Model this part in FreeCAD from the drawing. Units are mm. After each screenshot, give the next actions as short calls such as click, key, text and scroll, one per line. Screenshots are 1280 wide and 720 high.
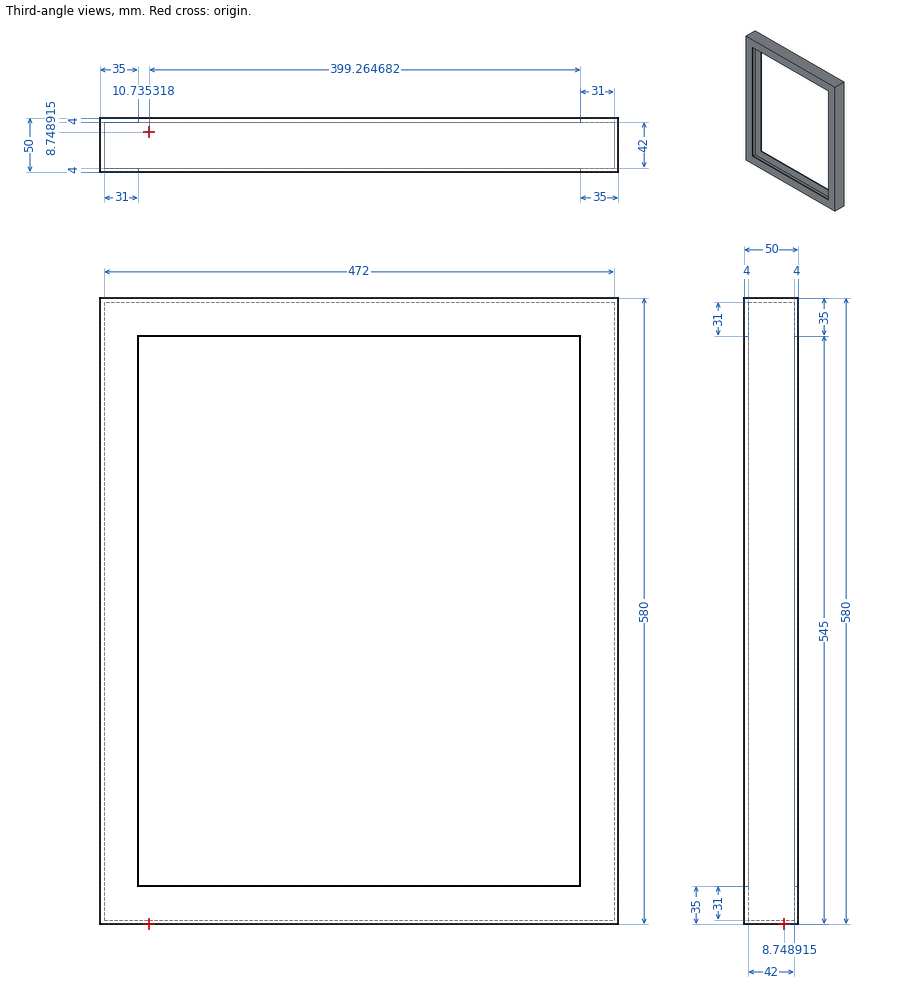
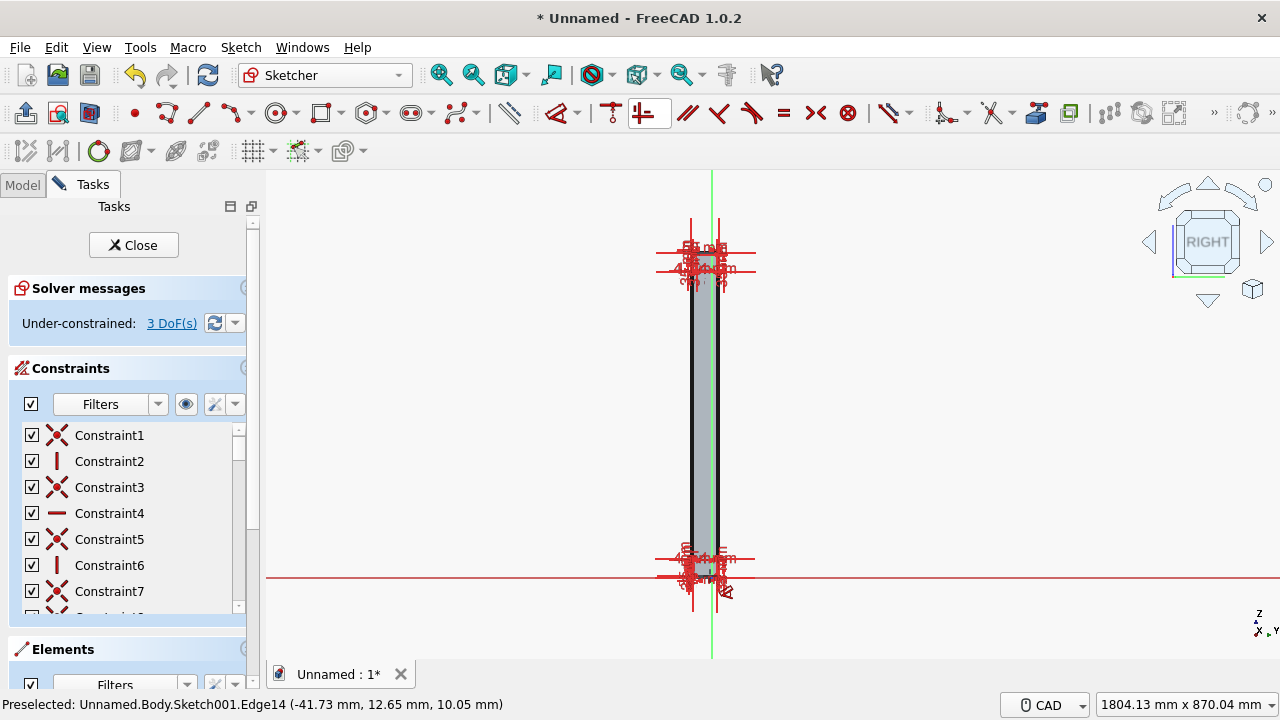
scroll(717, 272, up, 9)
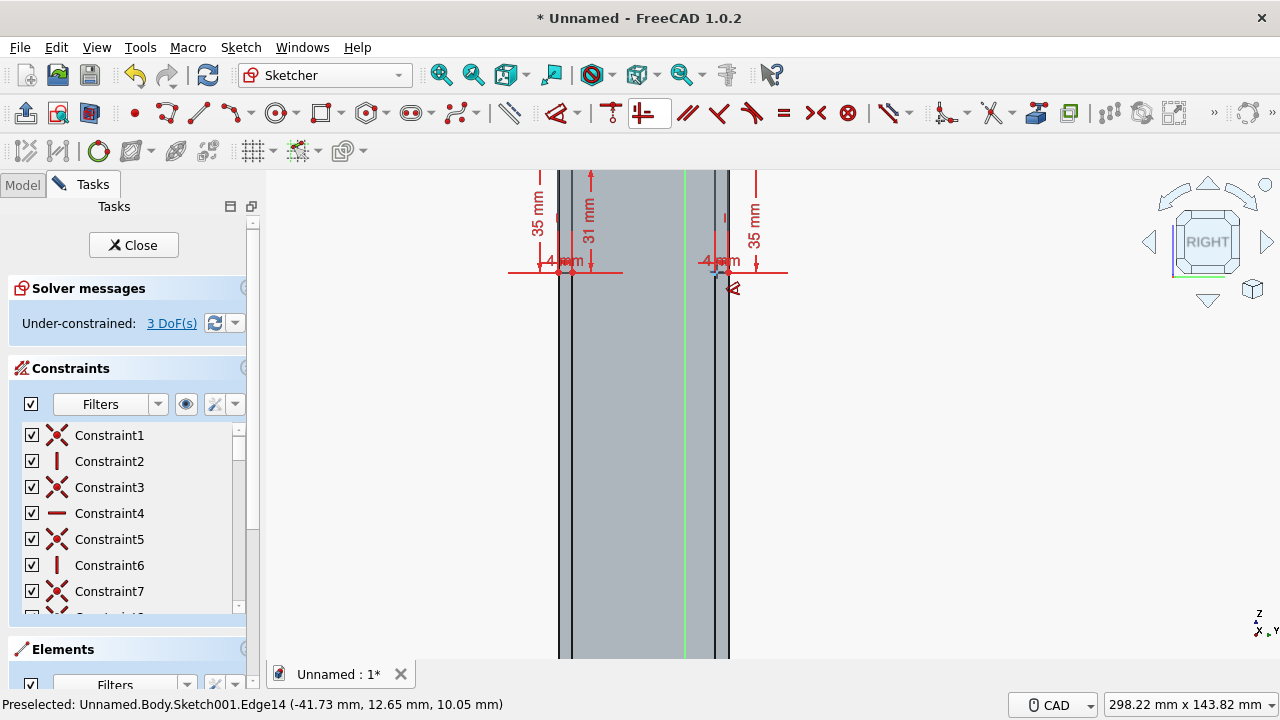
click(715, 273)
click(749, 452)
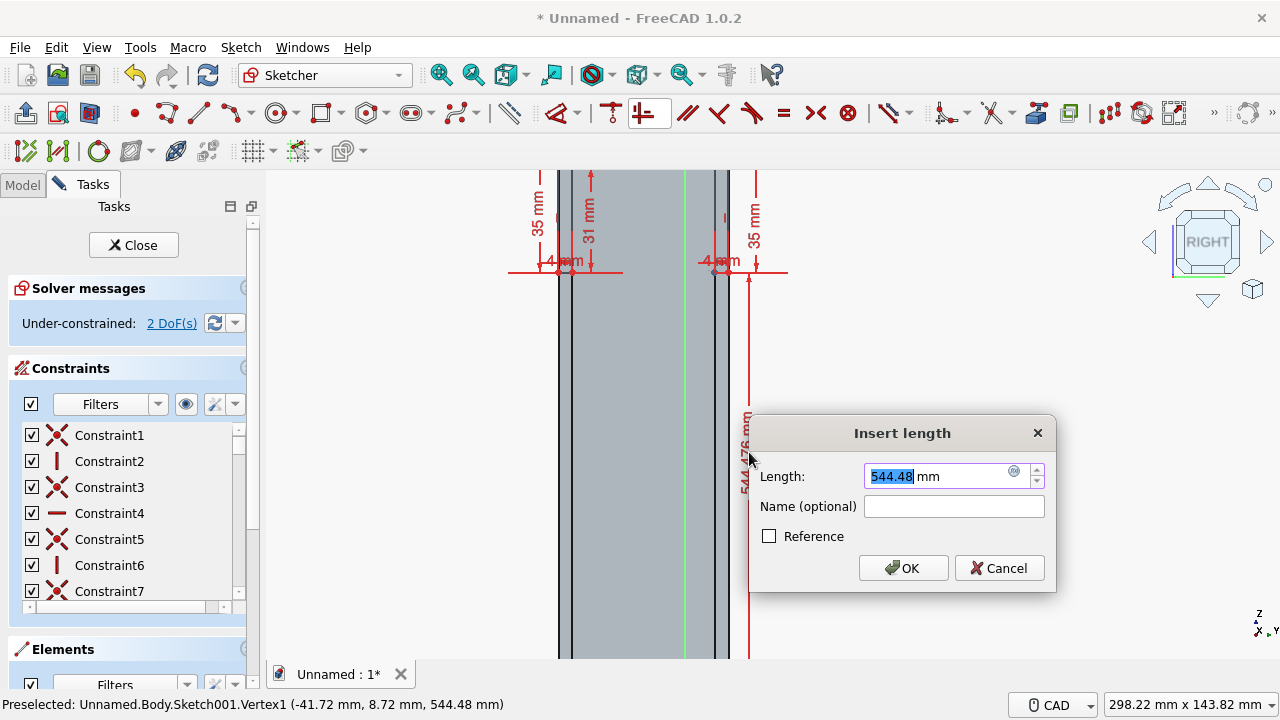
text(545)
key(Return)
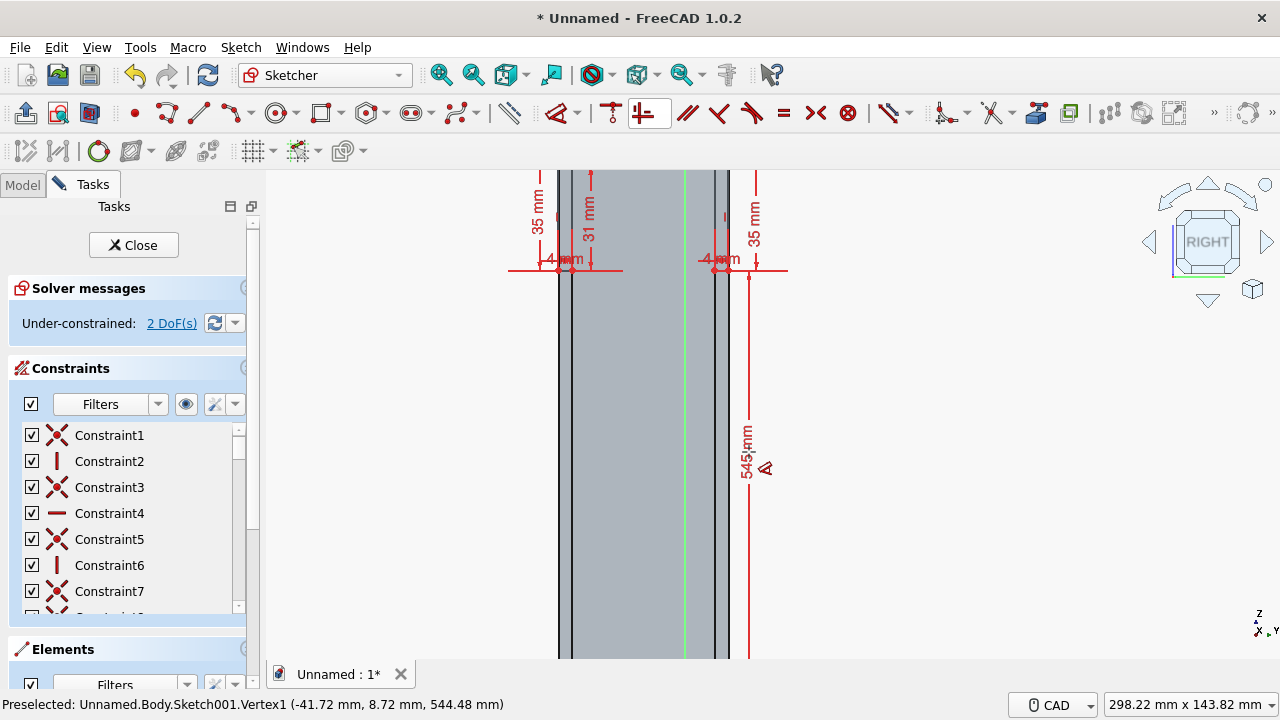
scroll(715, 271, up, 2)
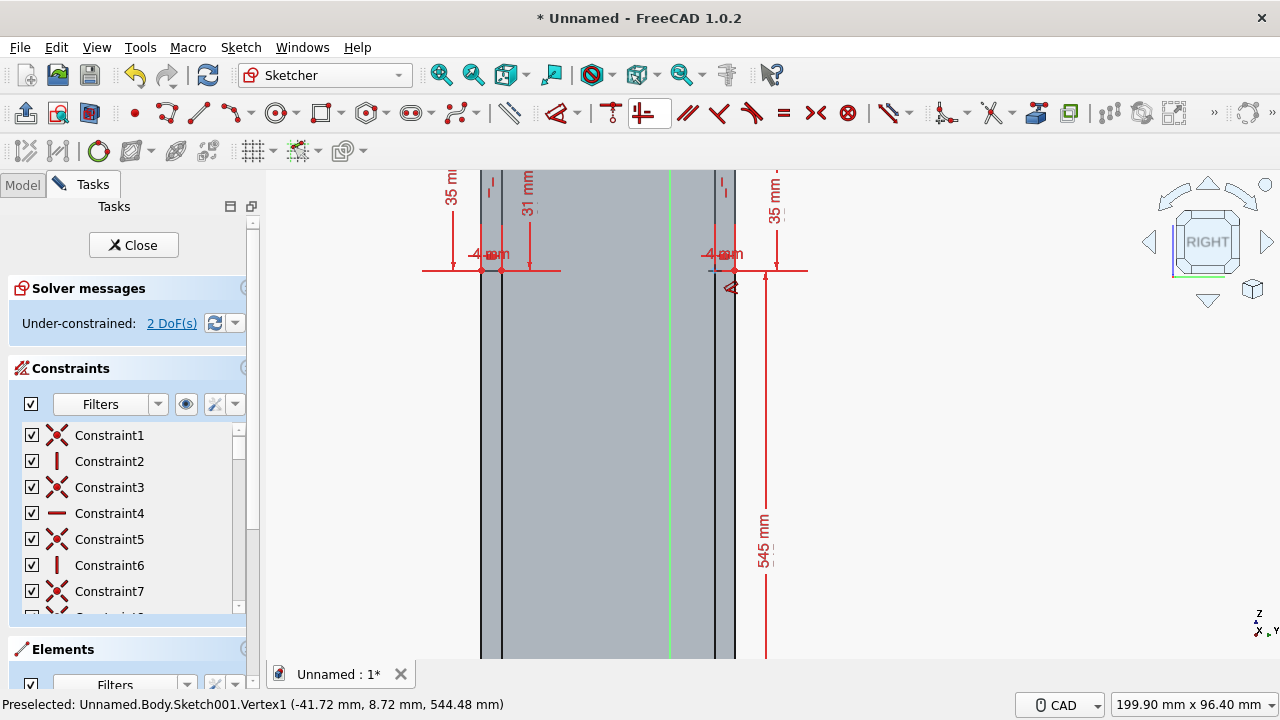
click(715, 271)
click(693, 237)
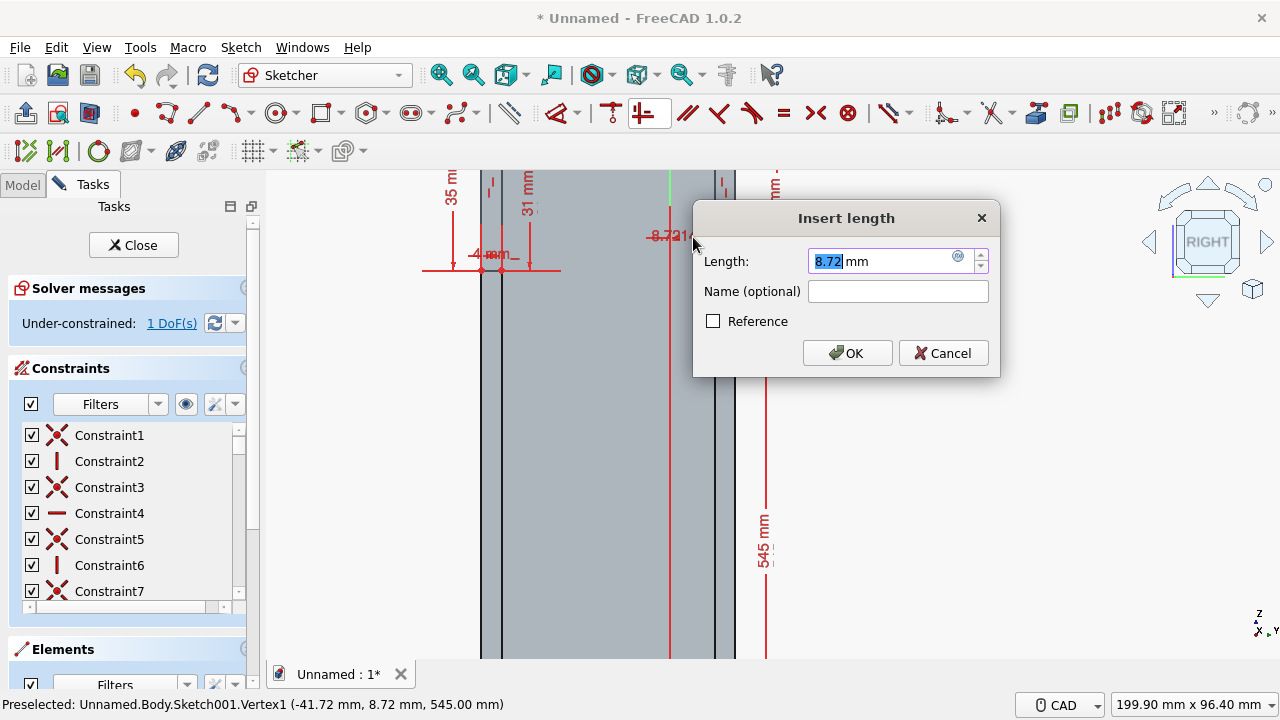
text(8.748915)
key(Return)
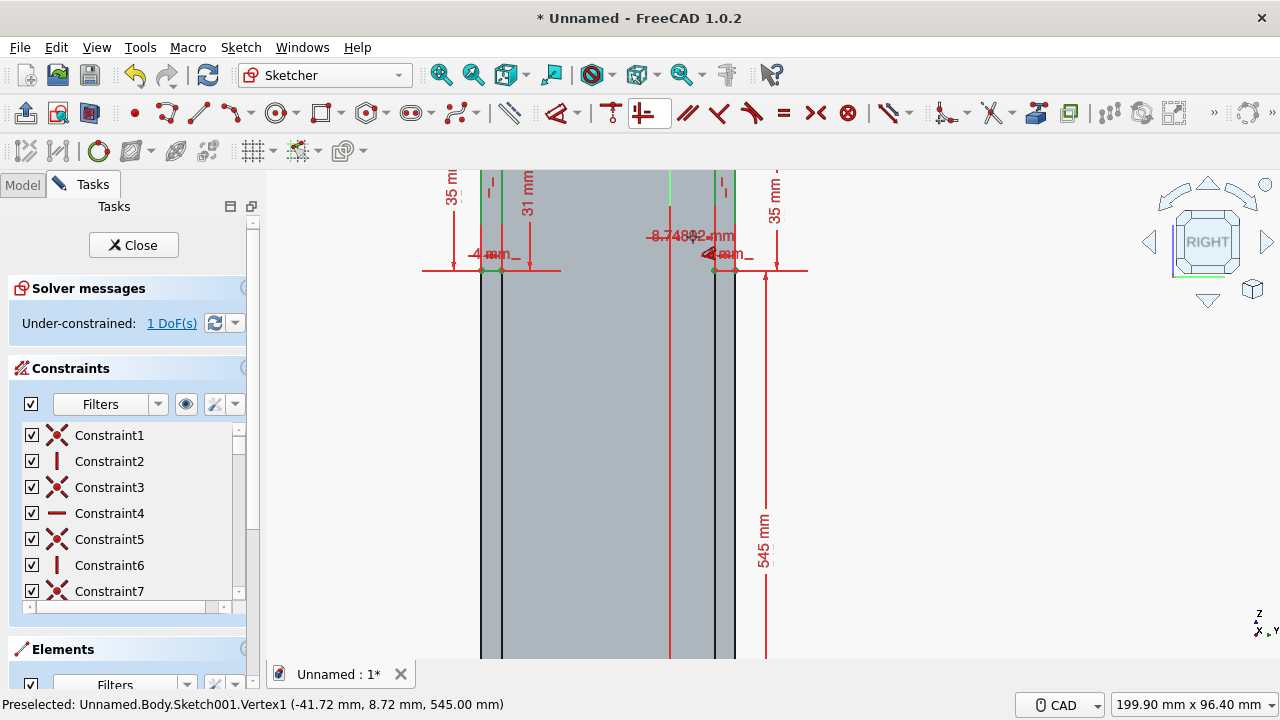
scroll(716, 271, down, 11)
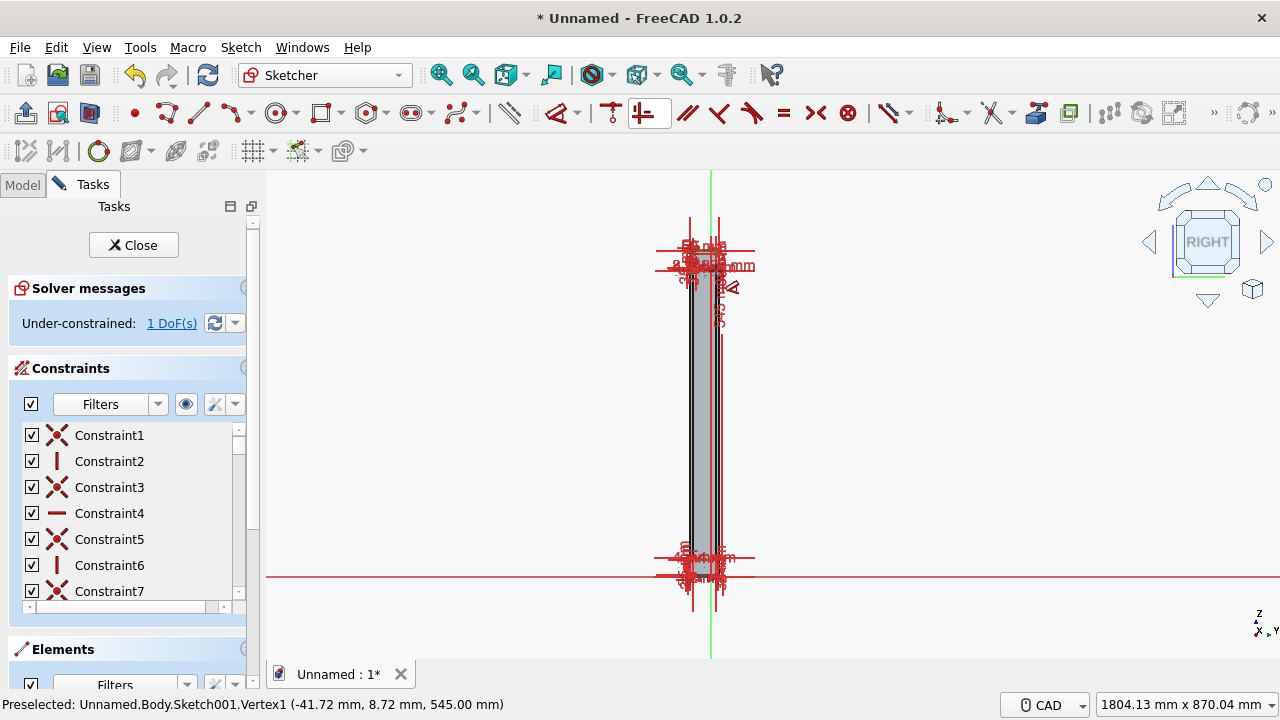
scroll(716, 575, up, 11)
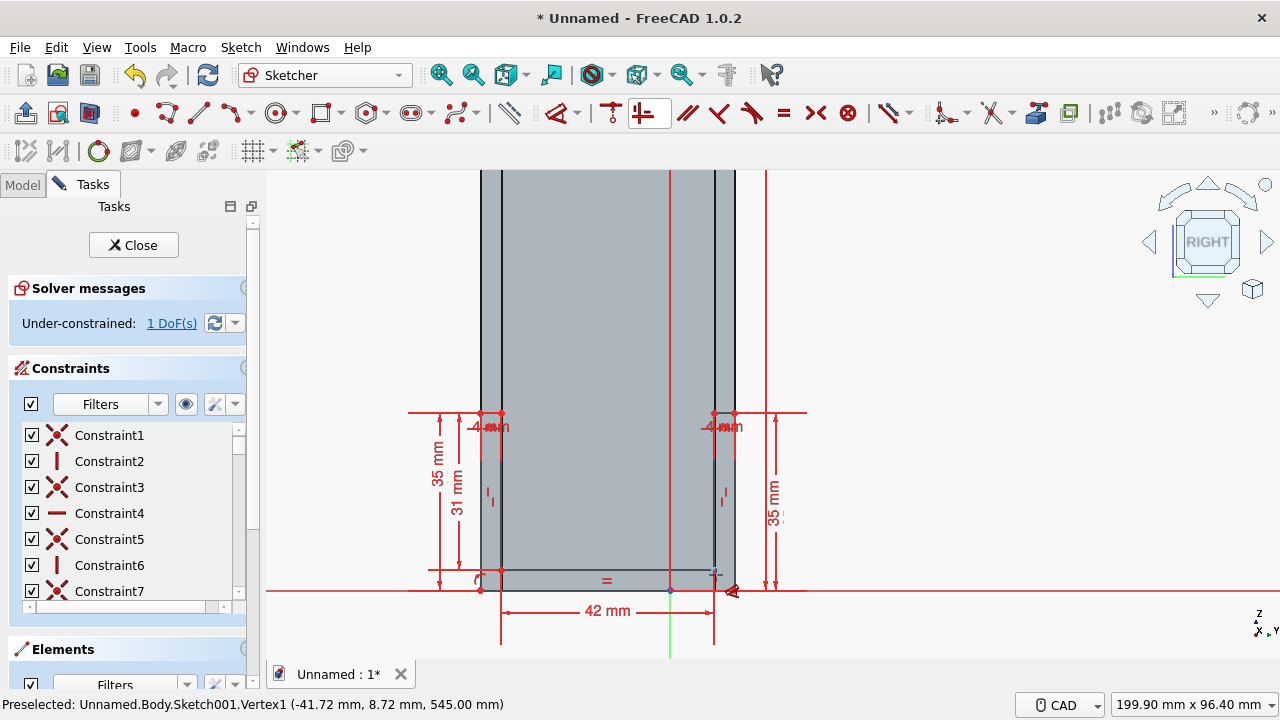
click(714, 570)
click(692, 625)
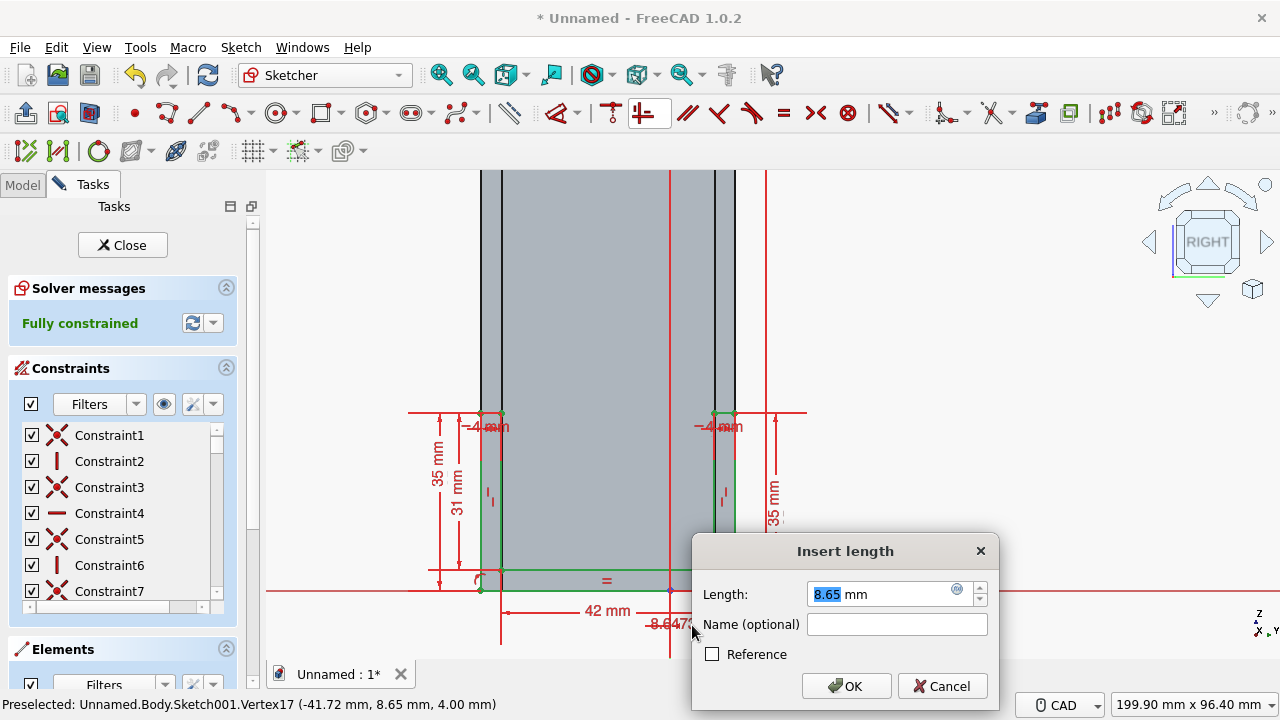
text(8.748915)
key(Return)
key(Escape)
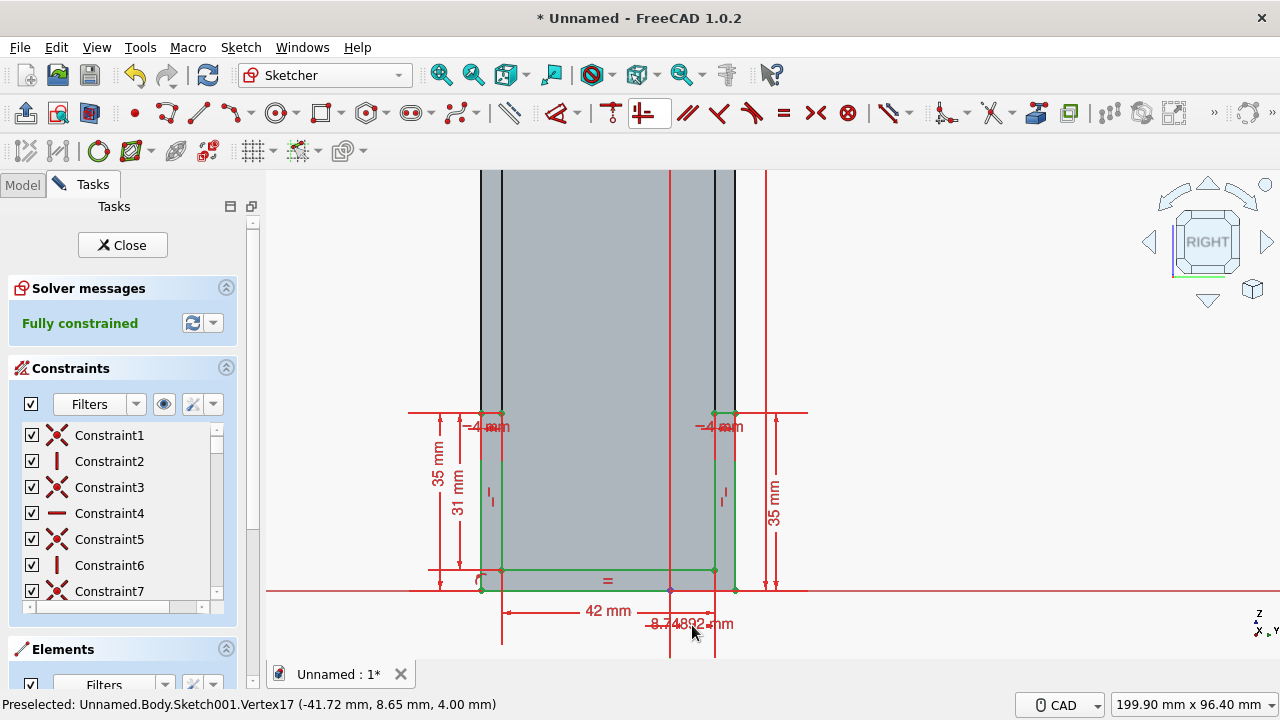
click(123, 245)